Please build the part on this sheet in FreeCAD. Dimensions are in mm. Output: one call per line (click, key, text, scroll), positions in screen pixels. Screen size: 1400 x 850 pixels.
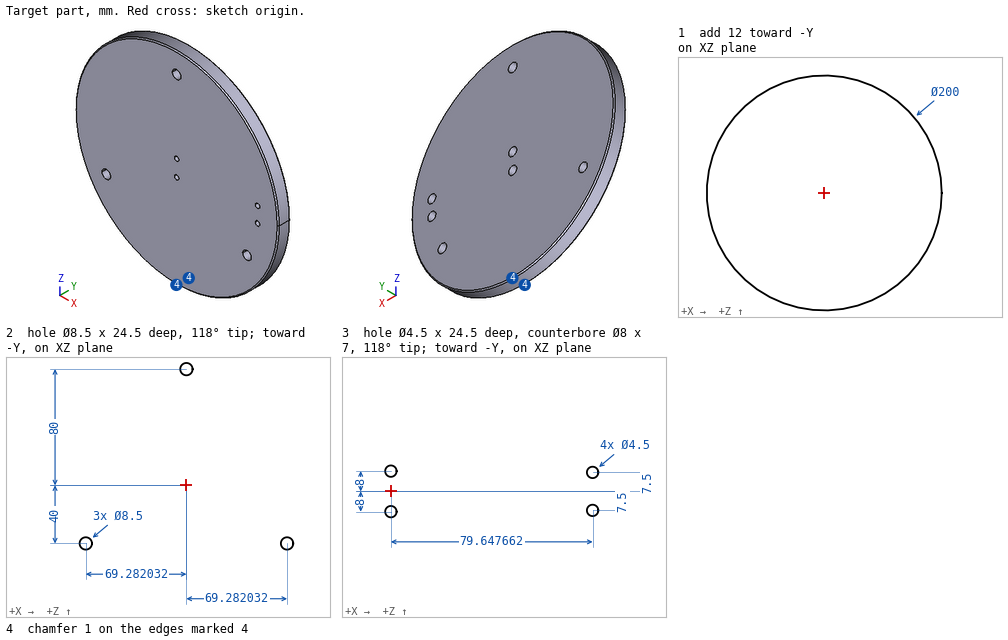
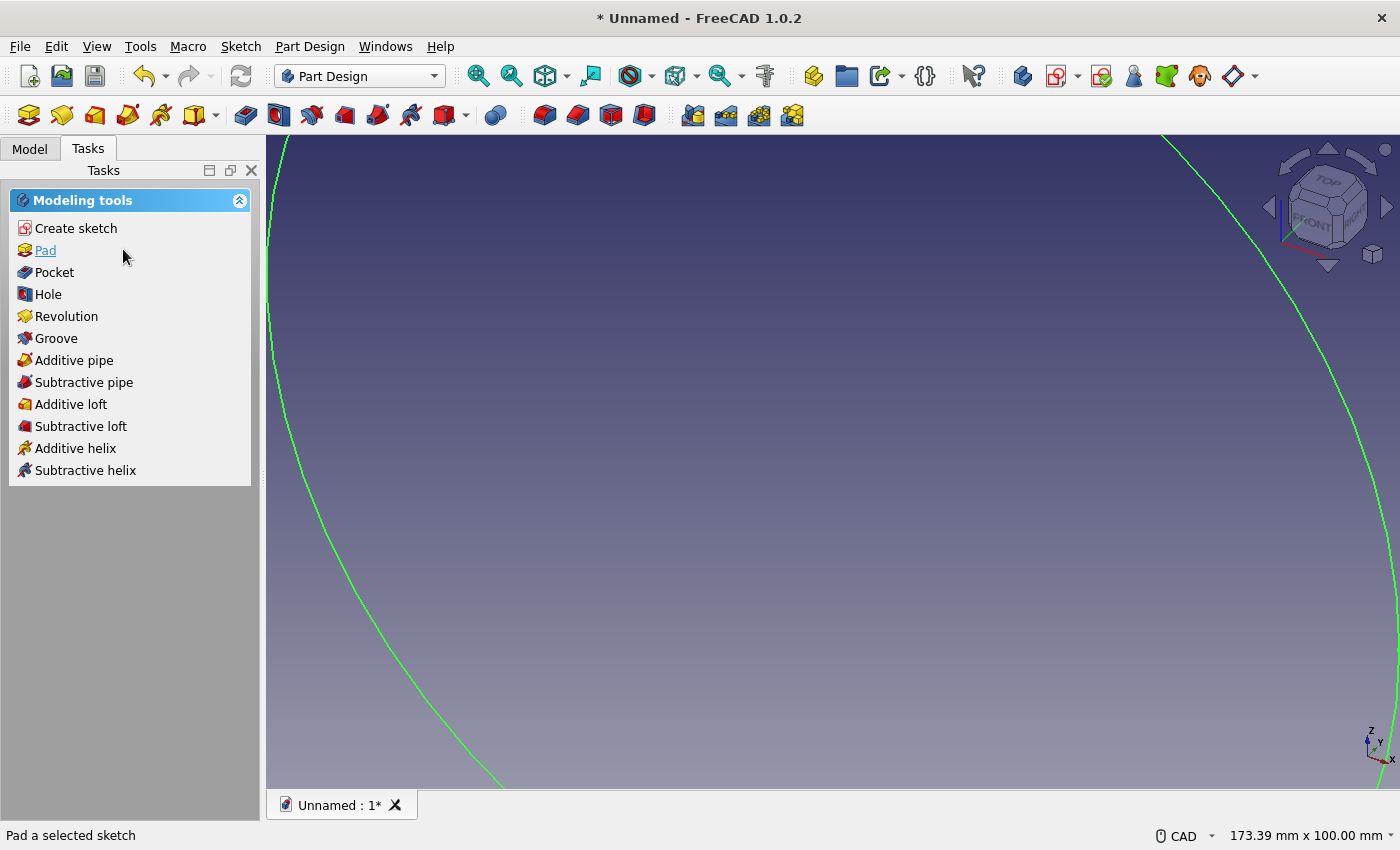
click(29, 116)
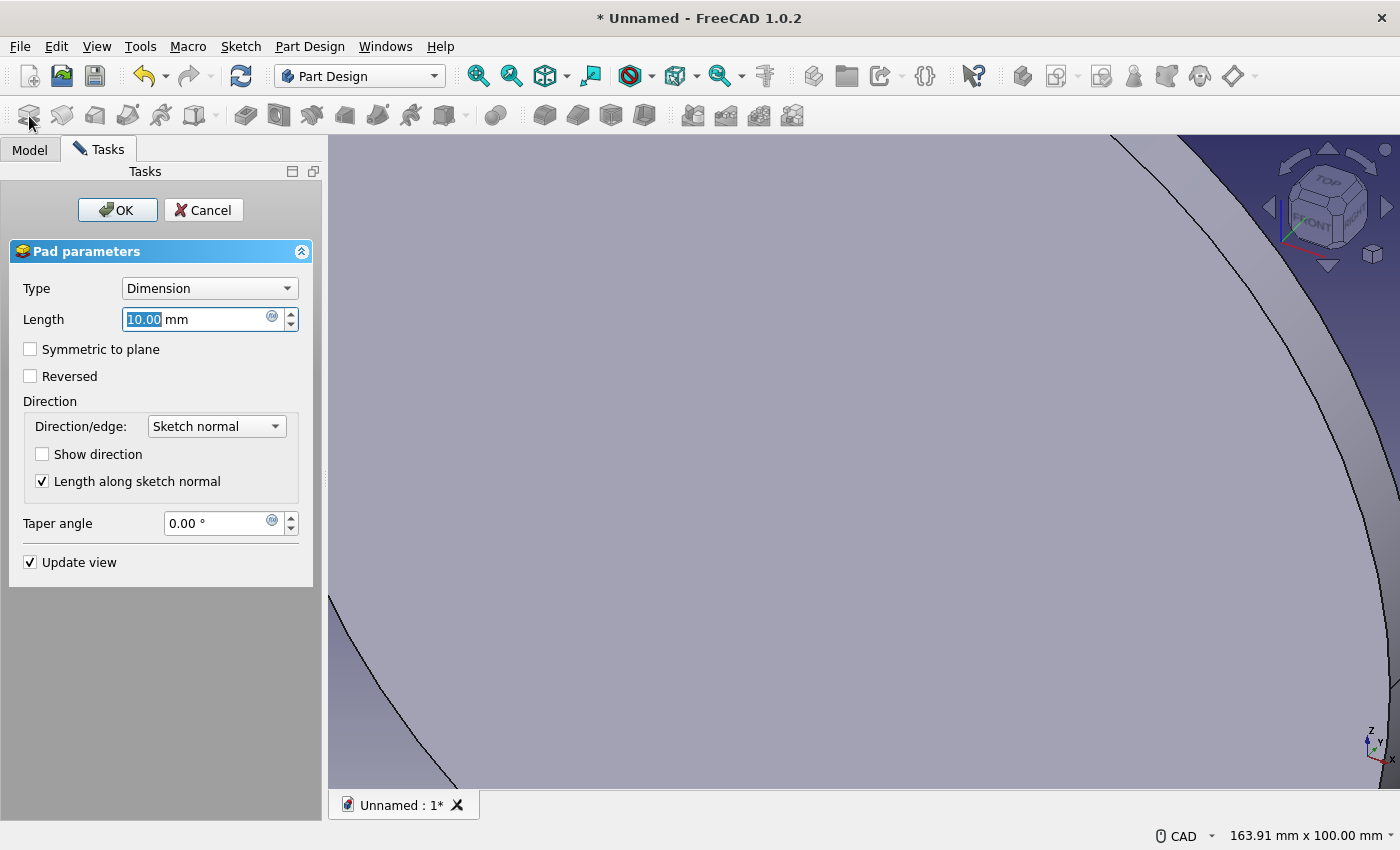
text(12)
key(Tab)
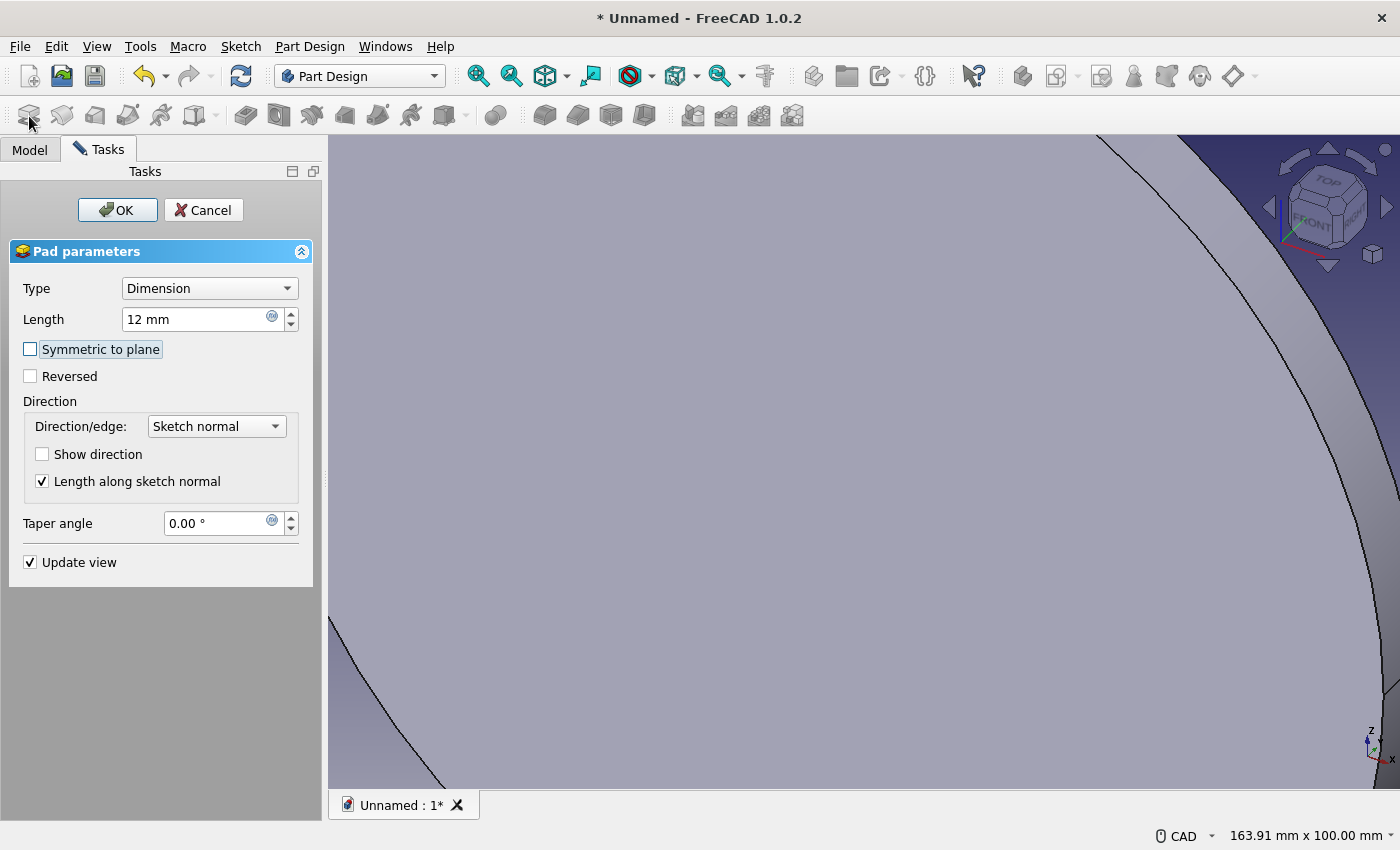
click(118, 210)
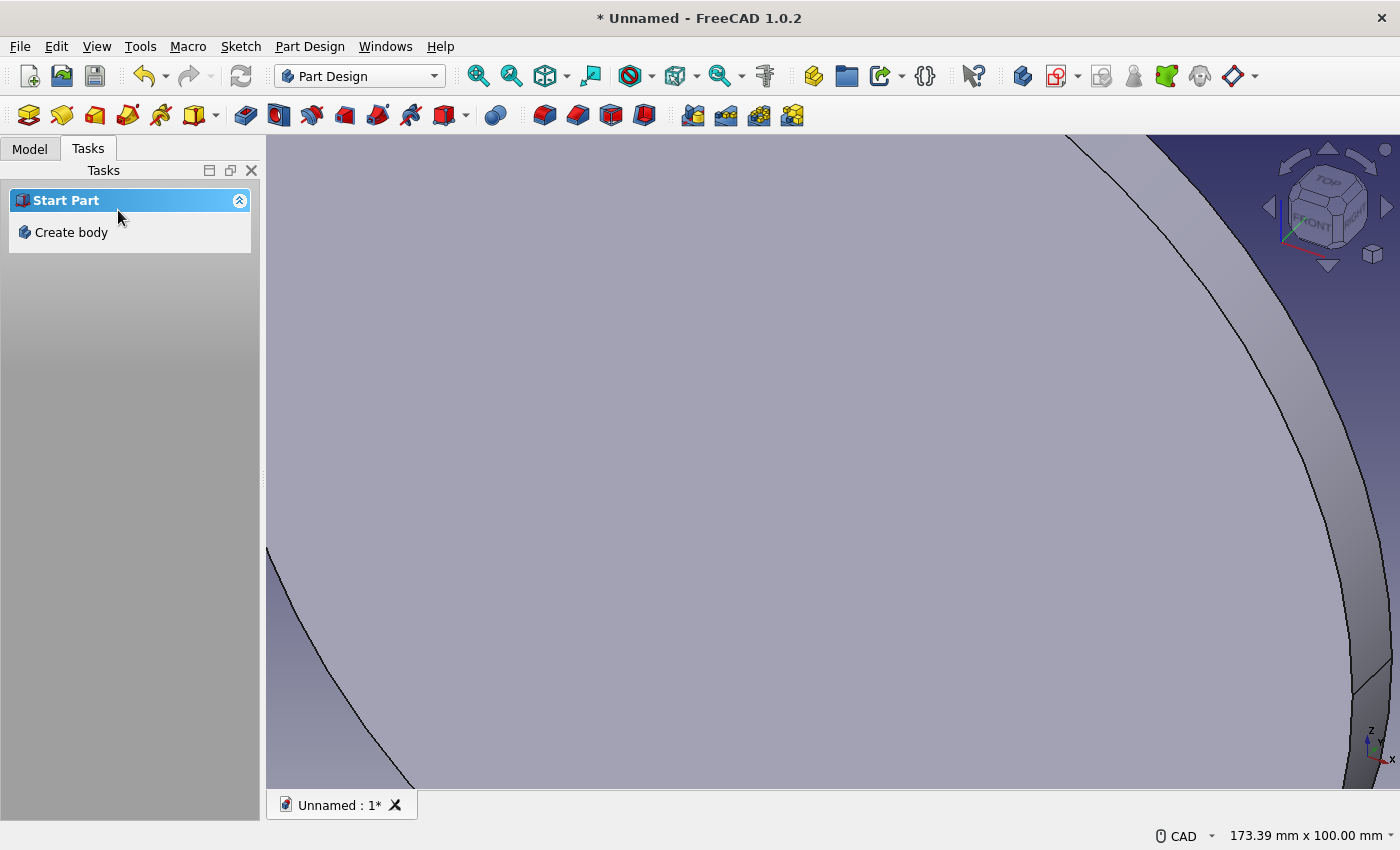
click(479, 76)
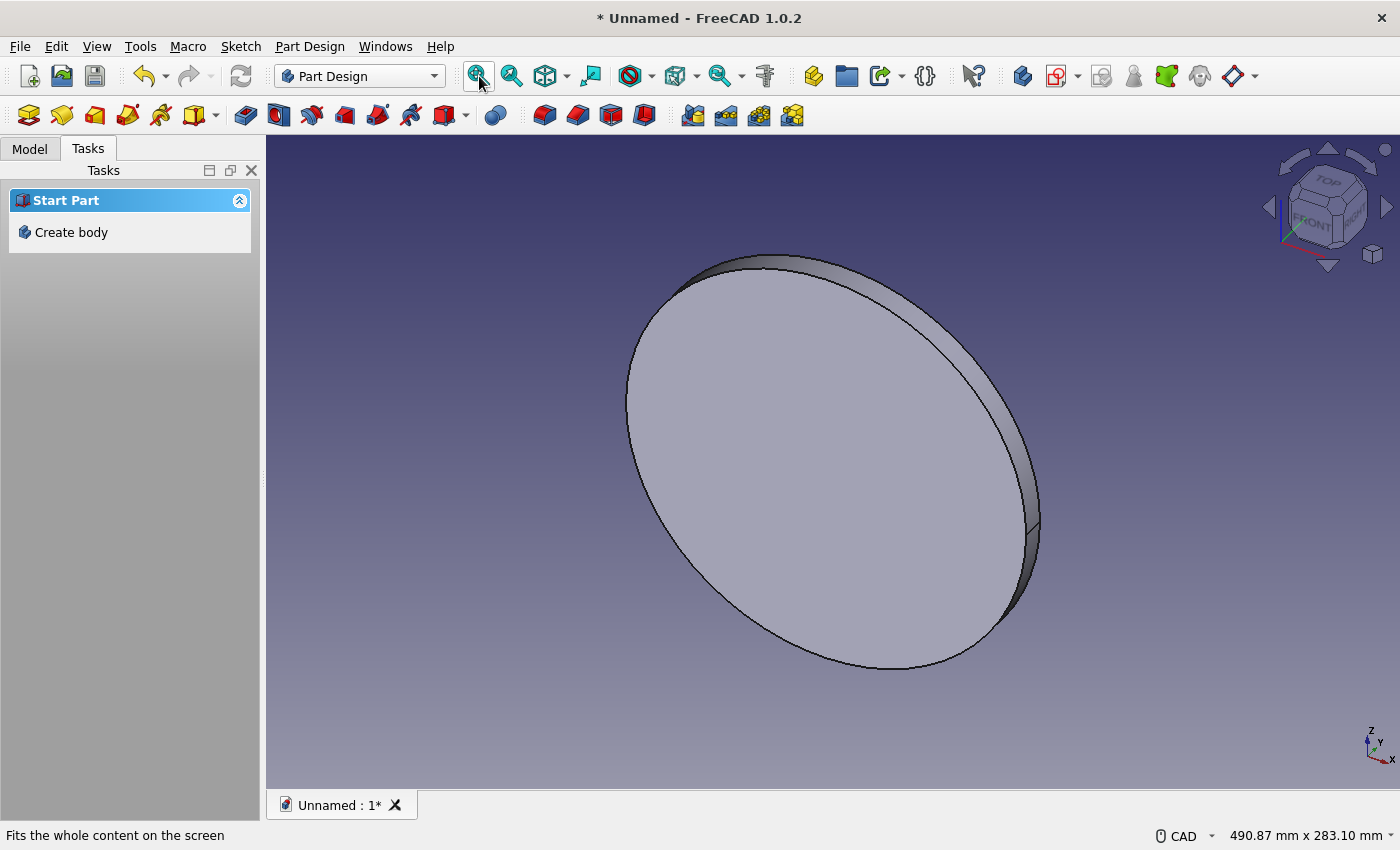
click(1056, 76)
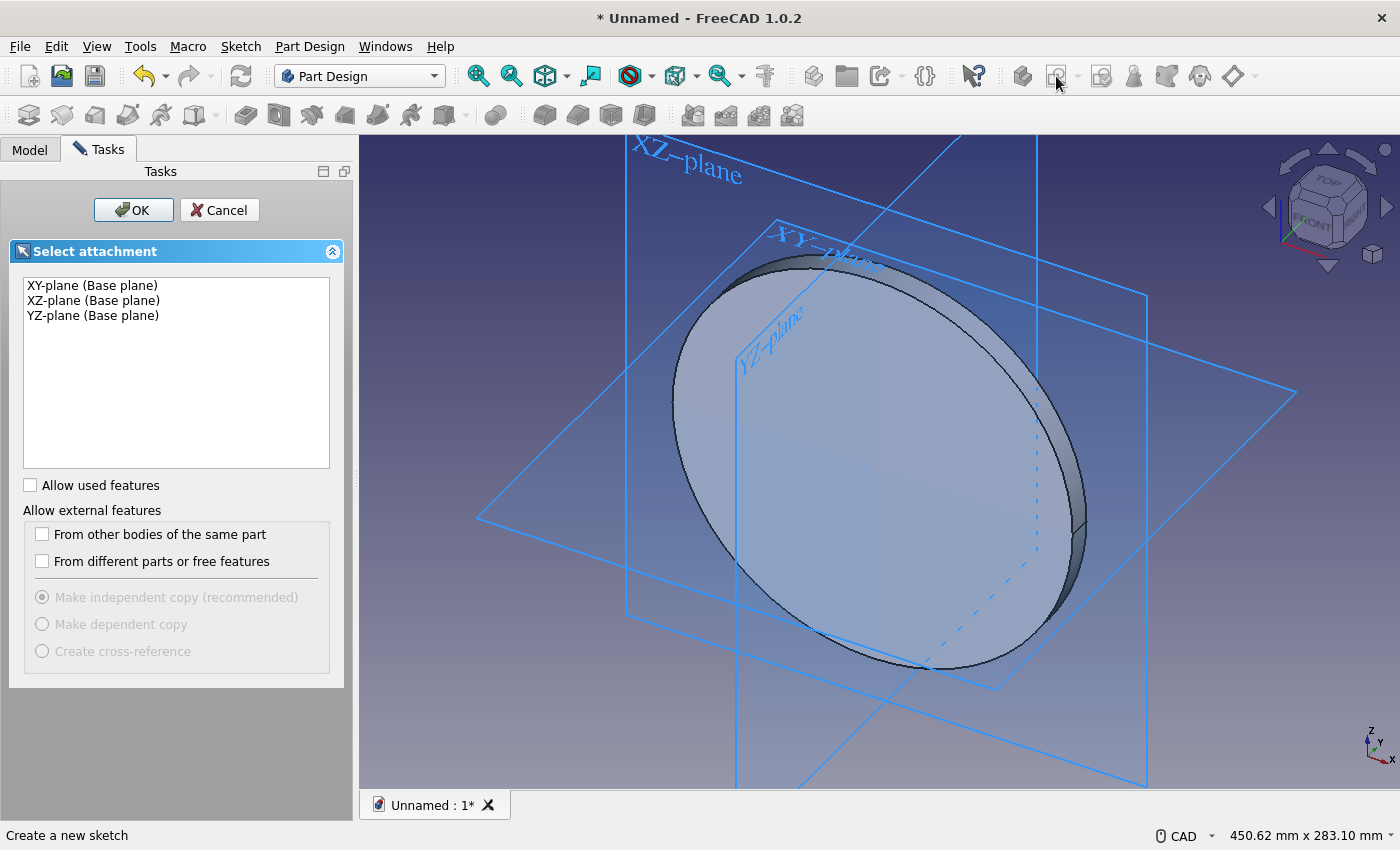
click(84, 300)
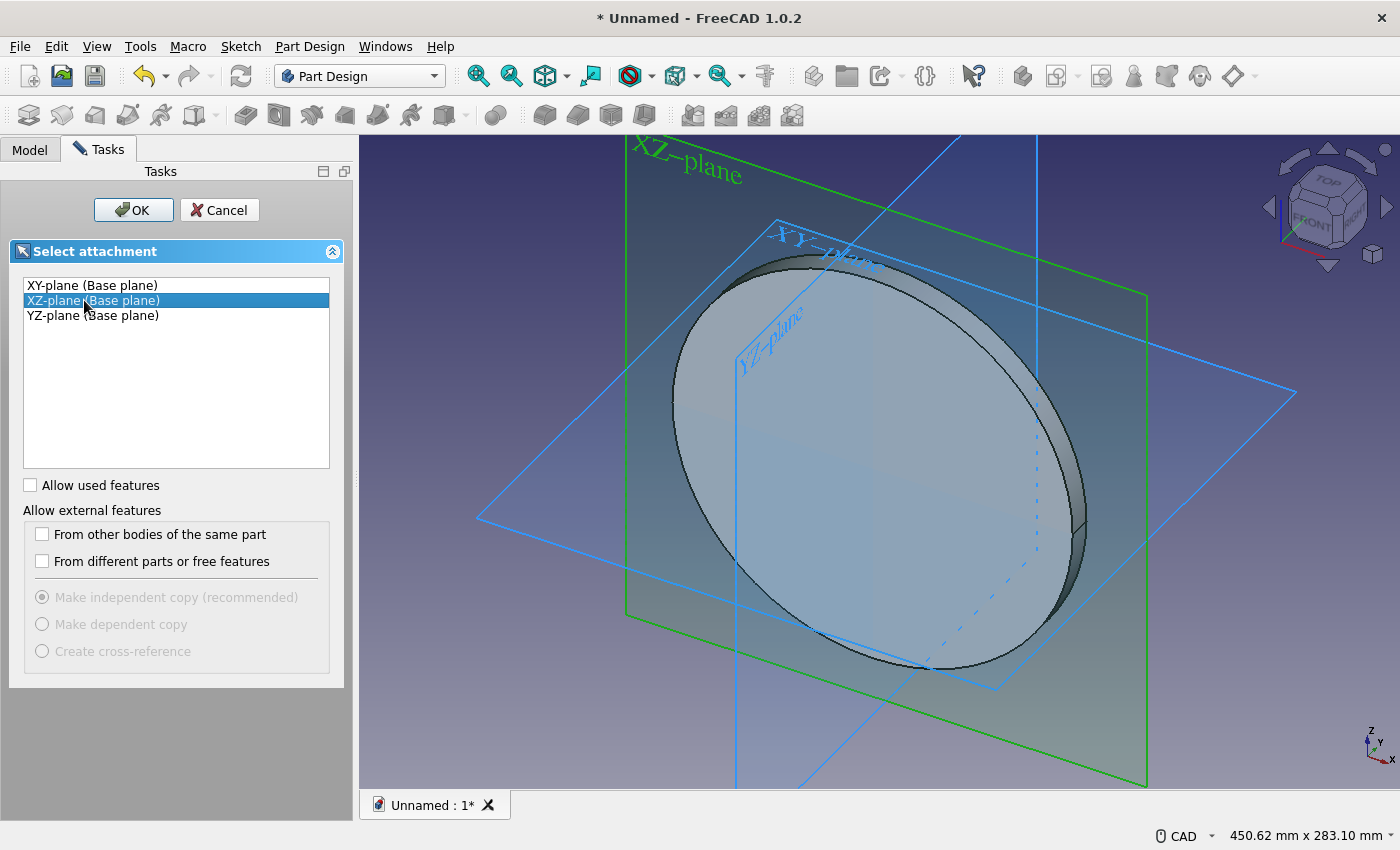
click(134, 210)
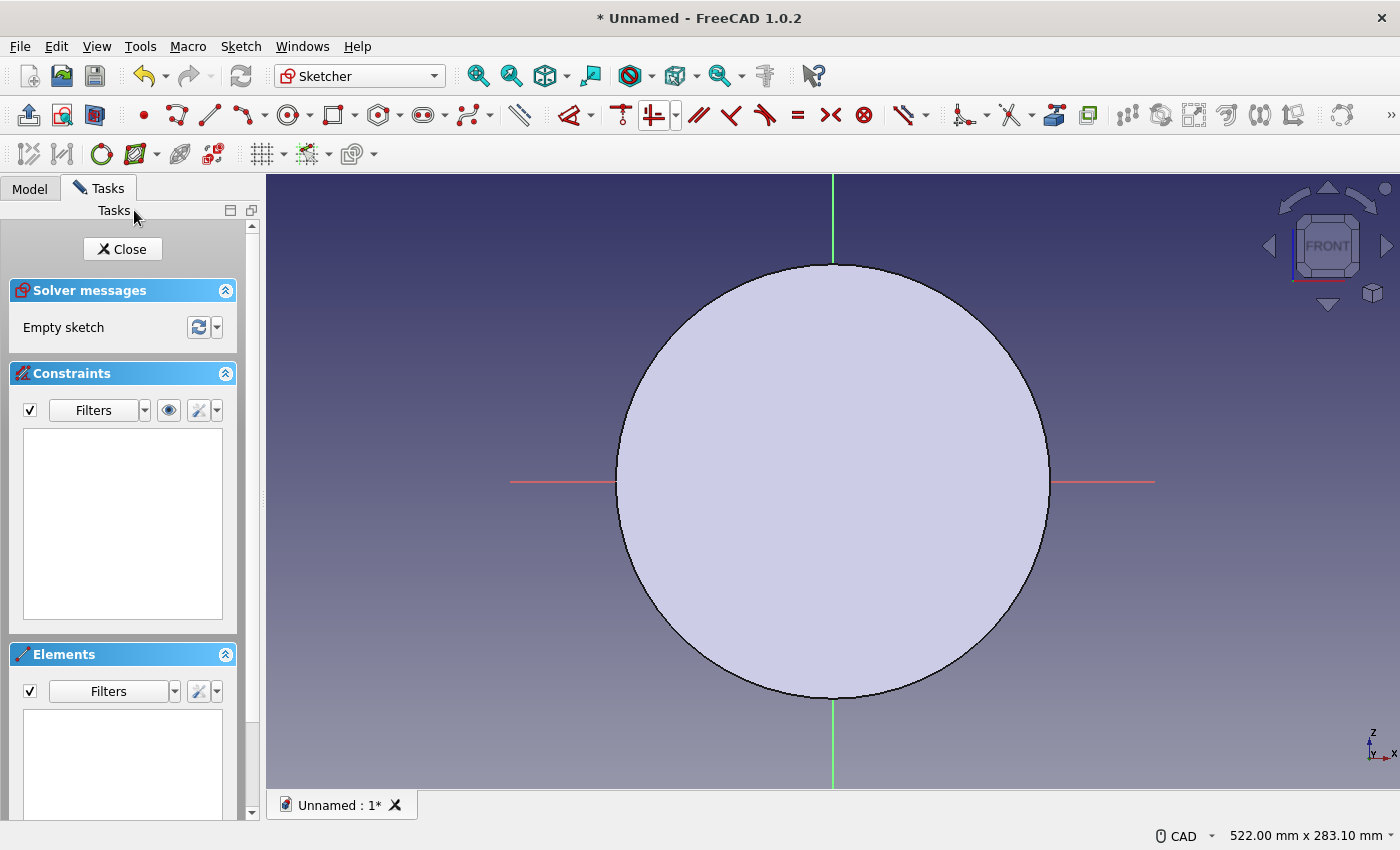
click(95, 116)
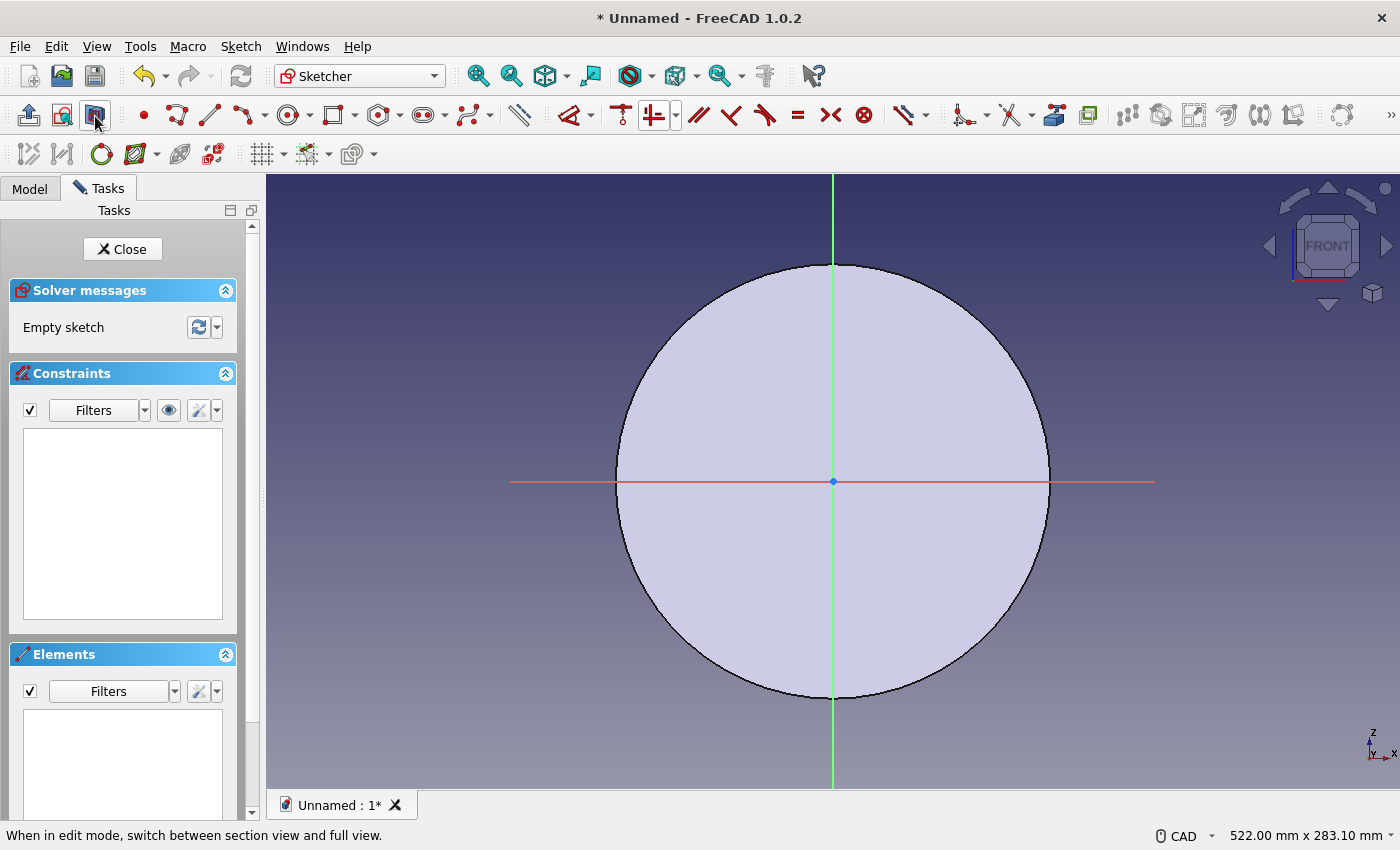
scroll(972, 350, up, 2)